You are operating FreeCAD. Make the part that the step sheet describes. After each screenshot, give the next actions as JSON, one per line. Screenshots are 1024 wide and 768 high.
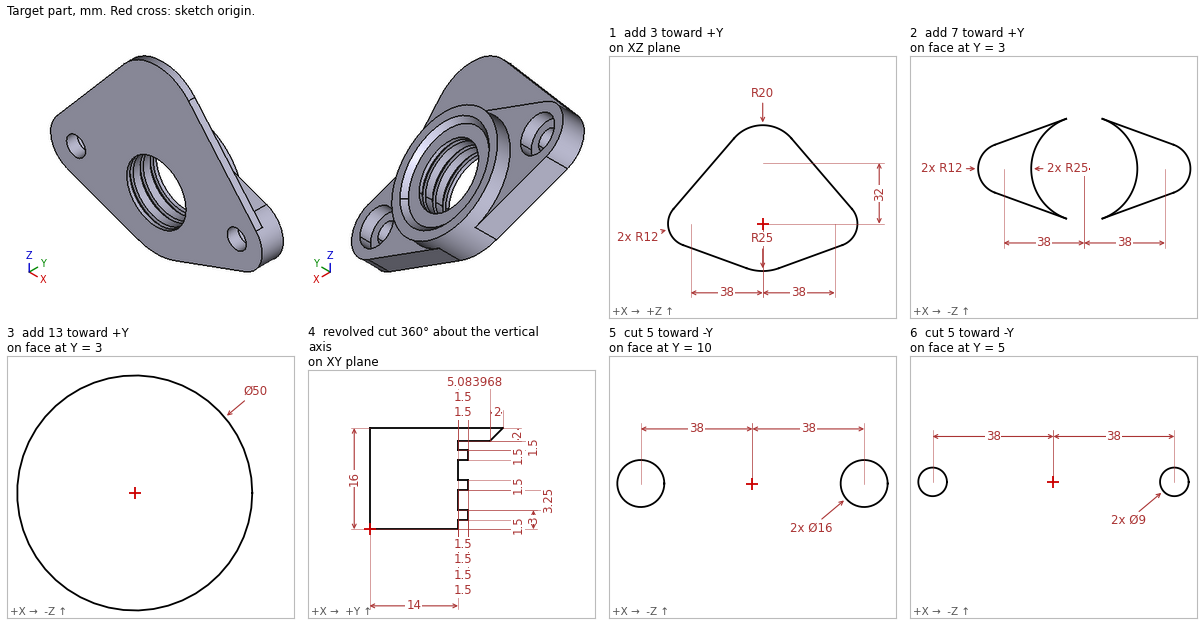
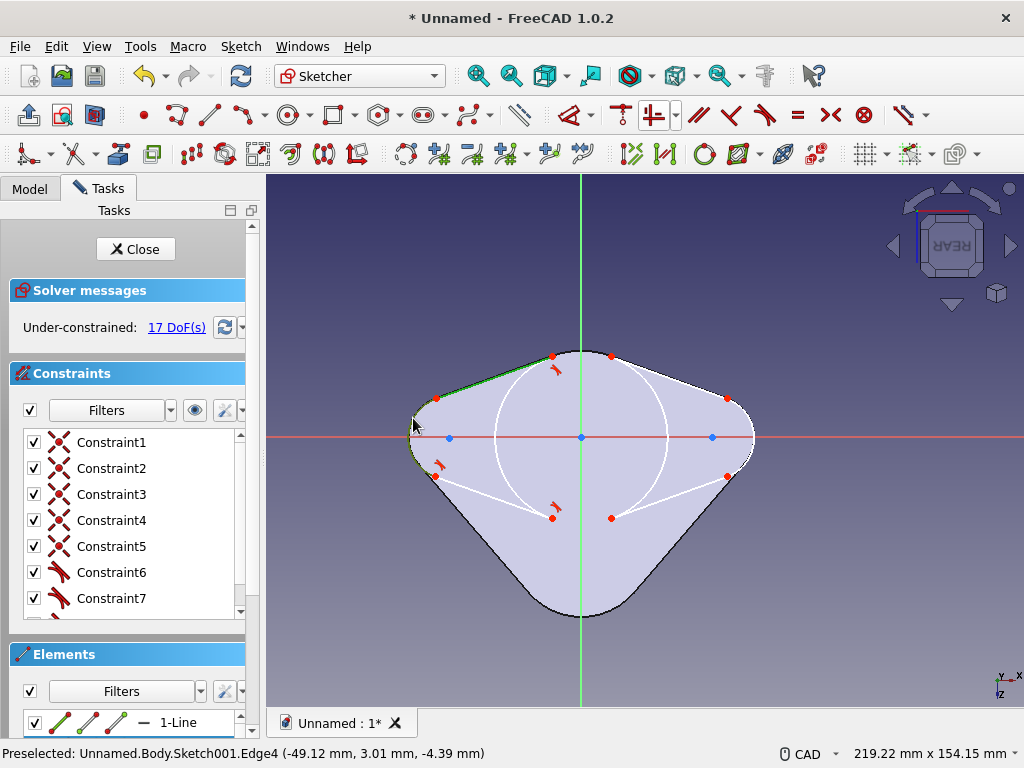
{"action": "left_click", "coordinate": [765, 116]}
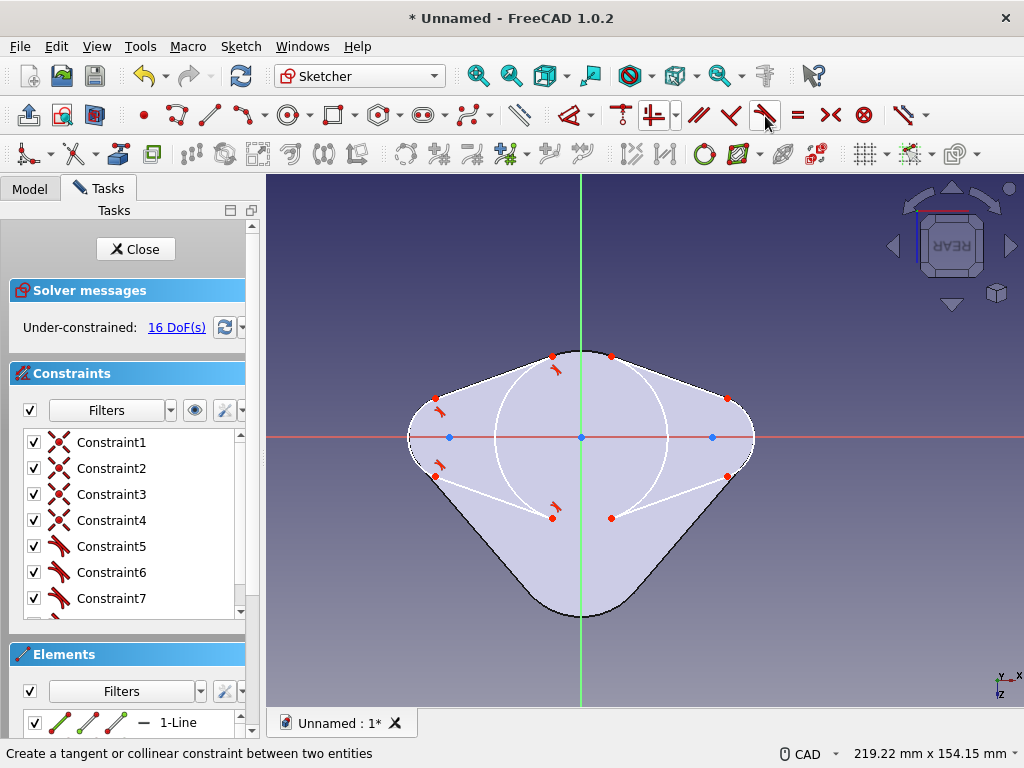
{"action": "left_click", "coordinate": [692, 490]}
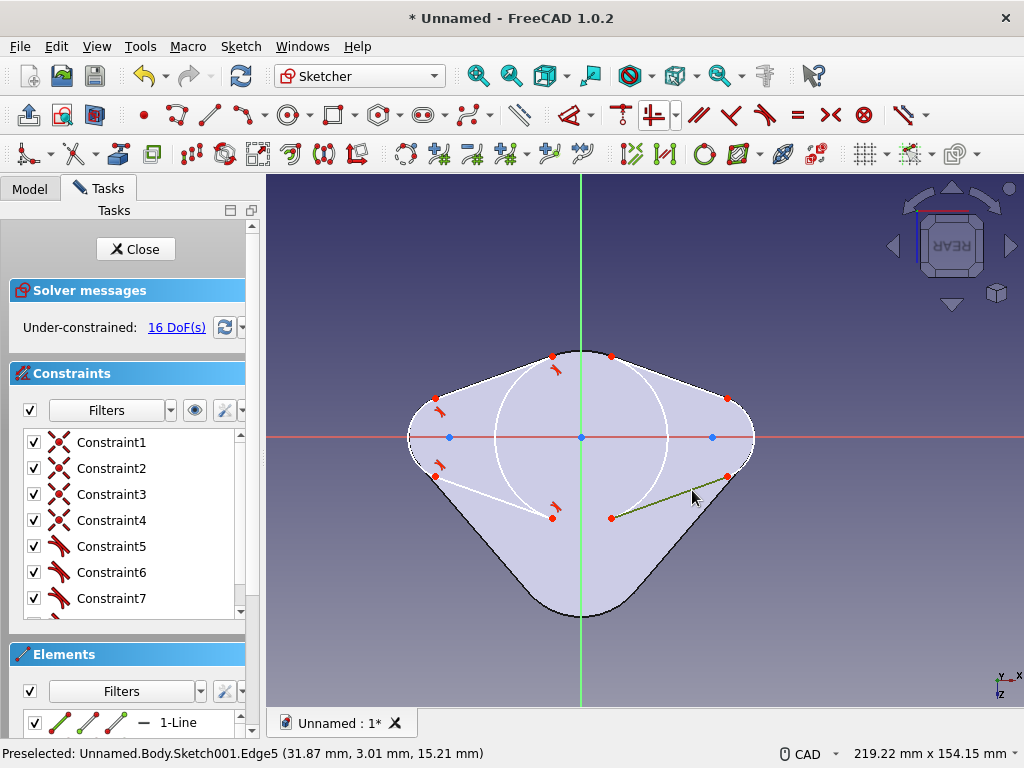
{"action": "left_click", "coordinate": [749, 457]}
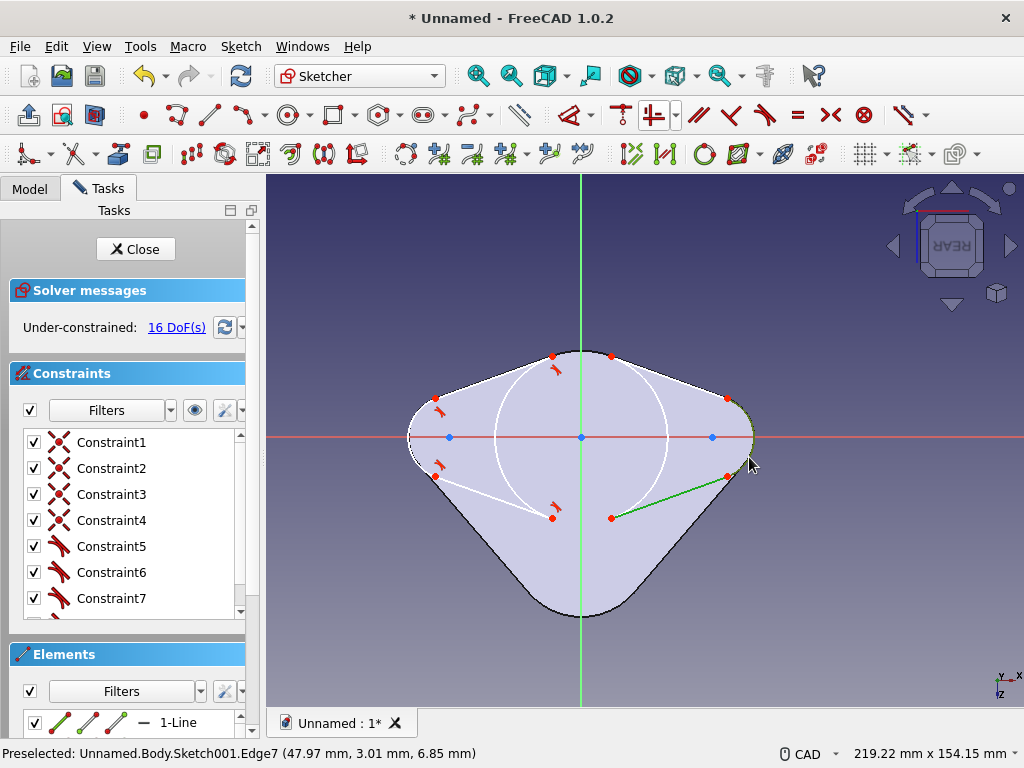
{"action": "left_click", "coordinate": [765, 116]}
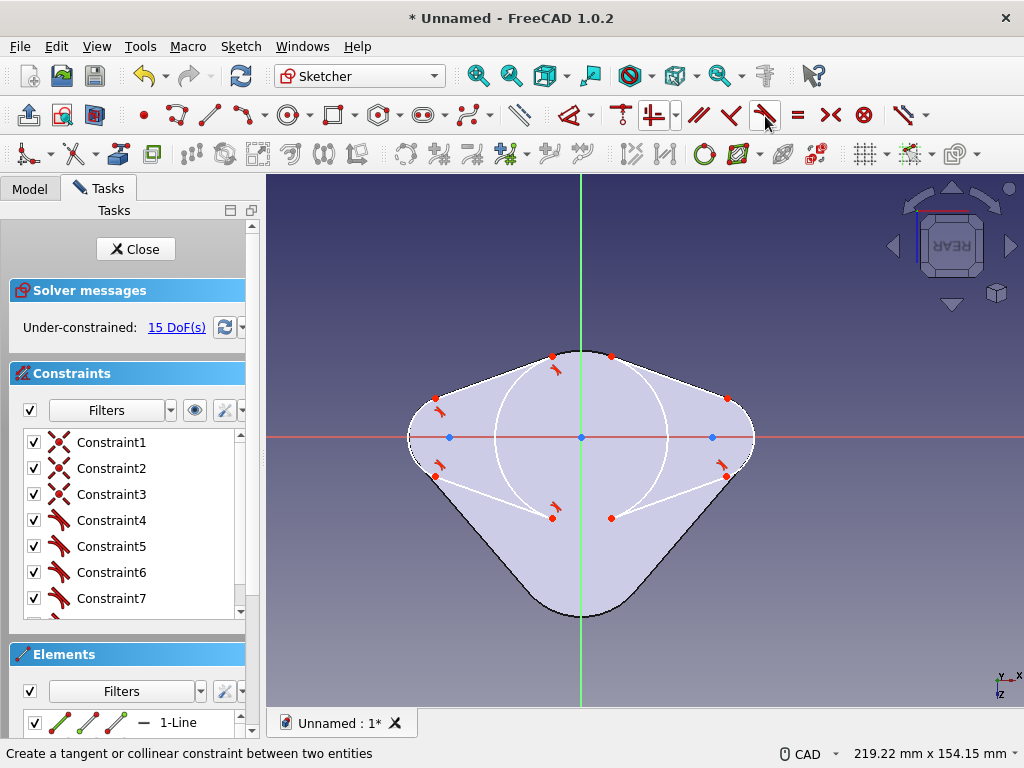
{"action": "left_click", "coordinate": [692, 490]}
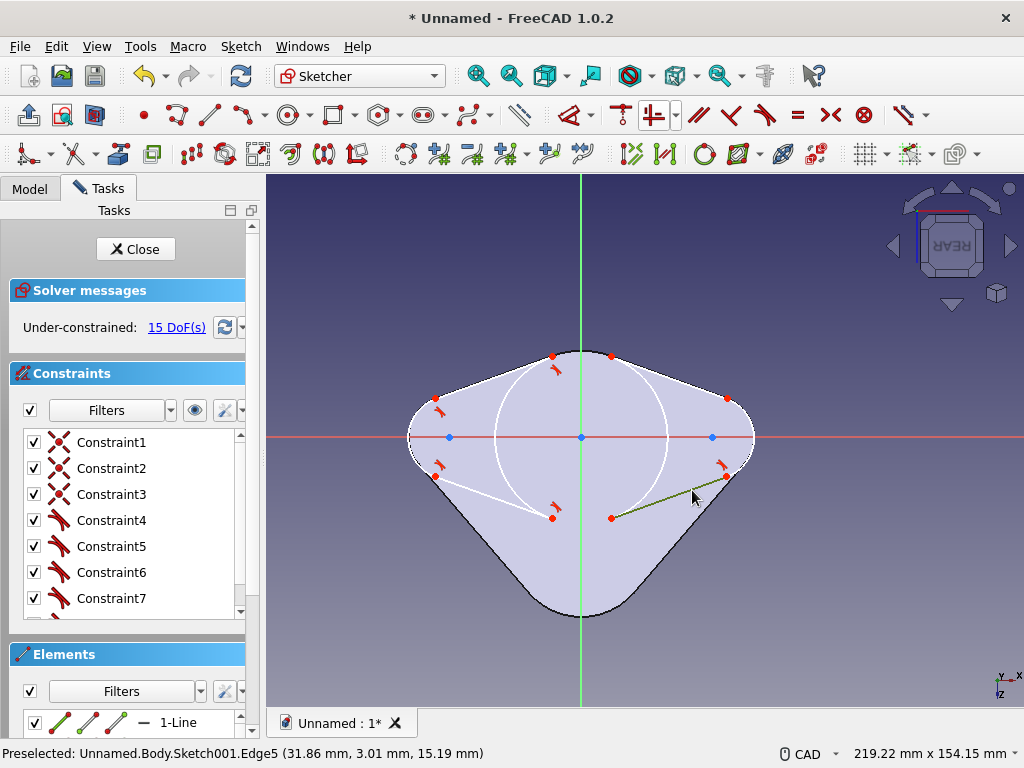
{"action": "left_click", "coordinate": [658, 478]}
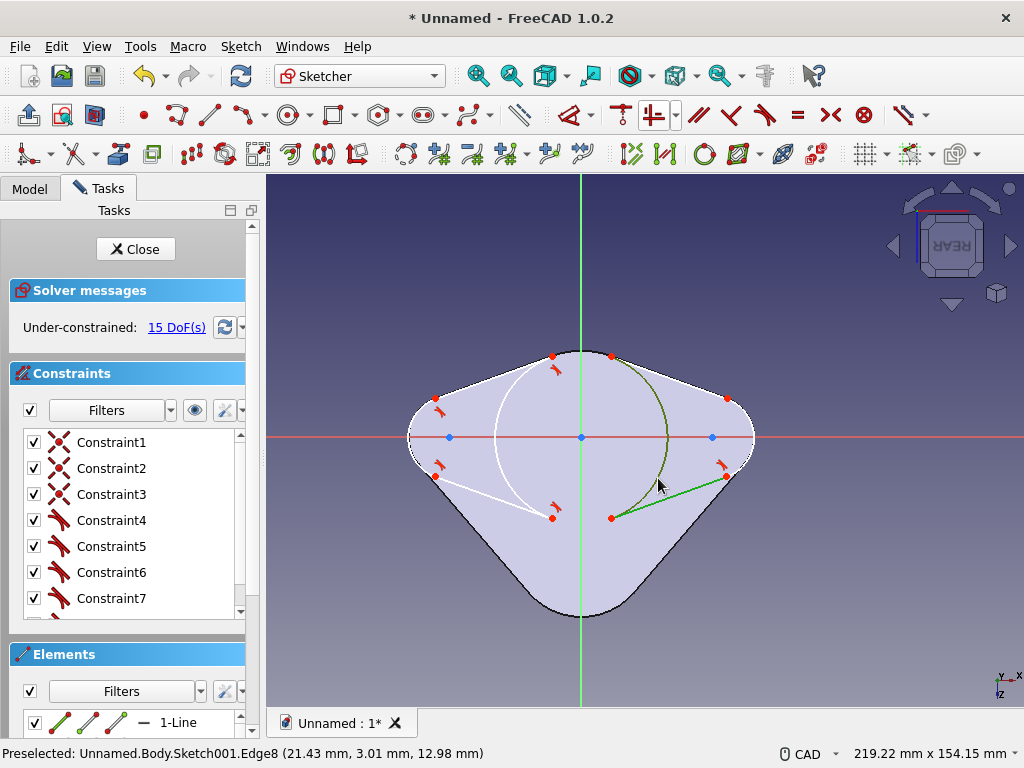
{"action": "left_click", "coordinate": [765, 116]}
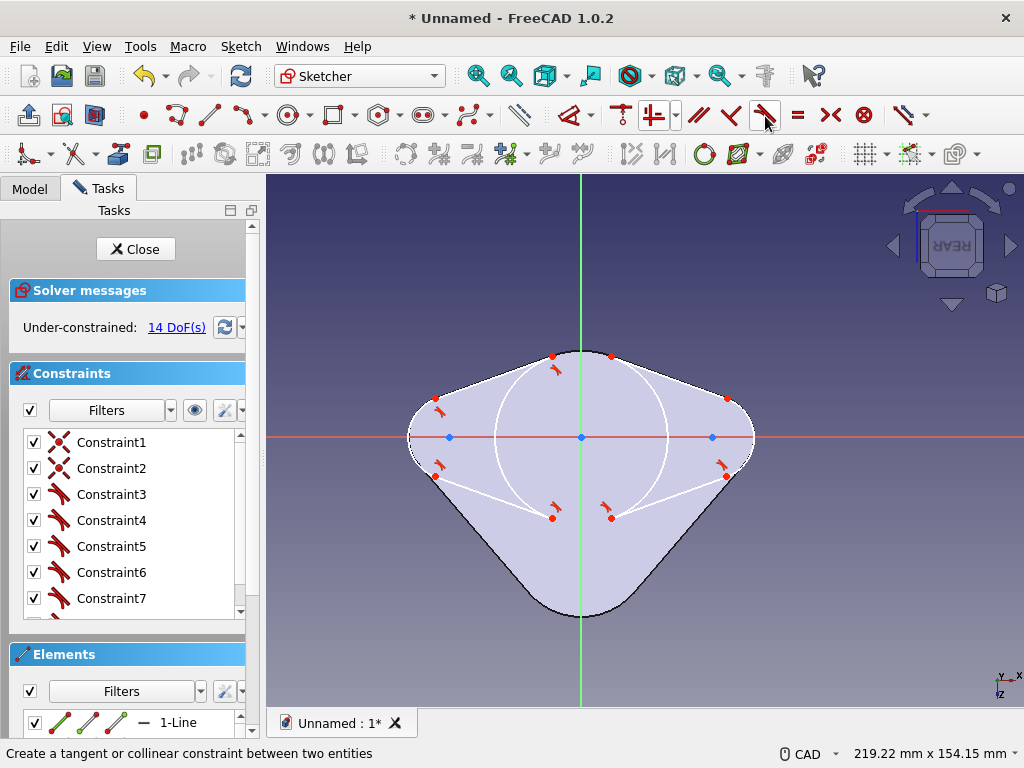
{"action": "left_click", "coordinate": [692, 386]}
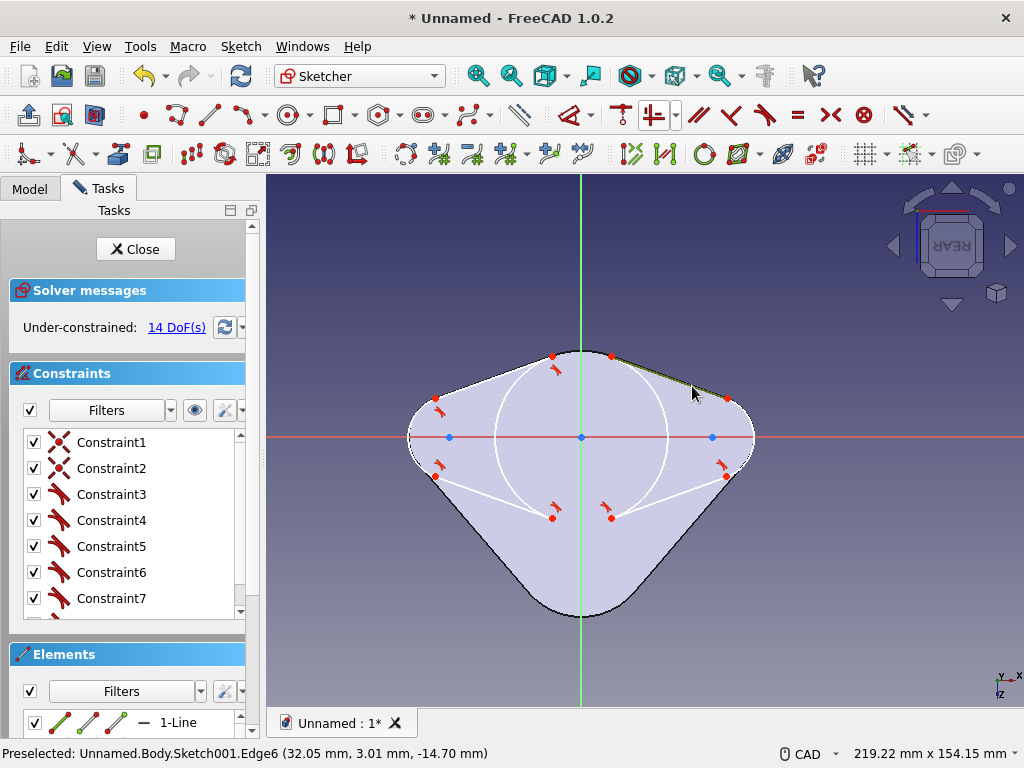
{"action": "left_click", "coordinate": [749, 458]}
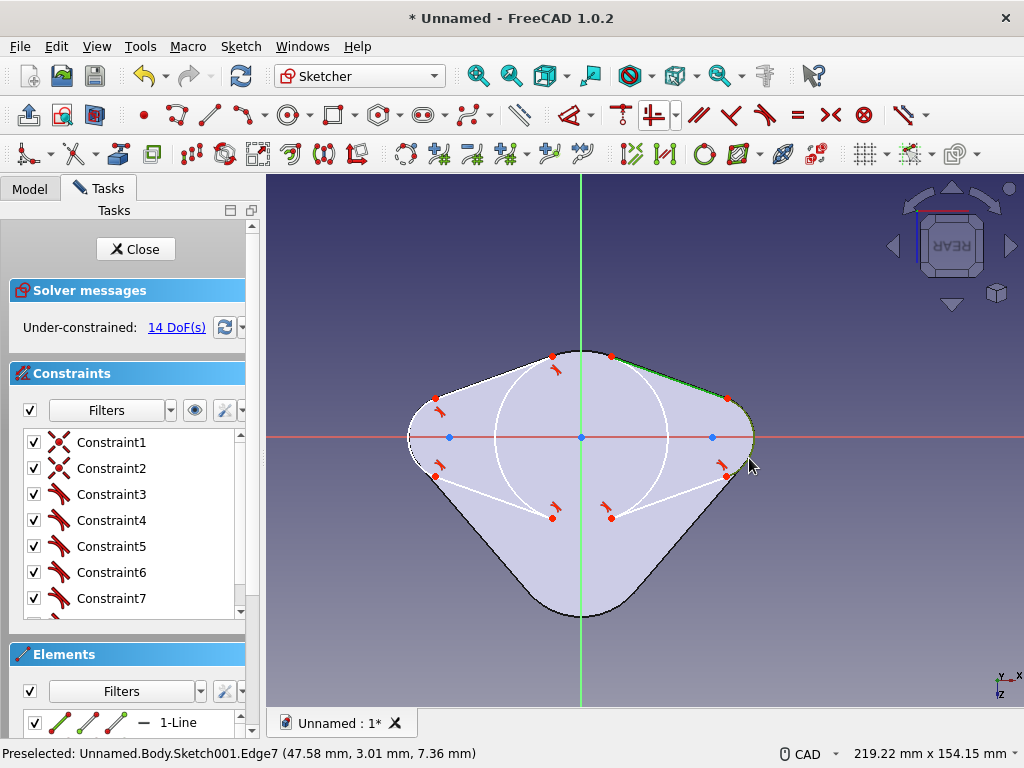
{"action": "left_click", "coordinate": [765, 116]}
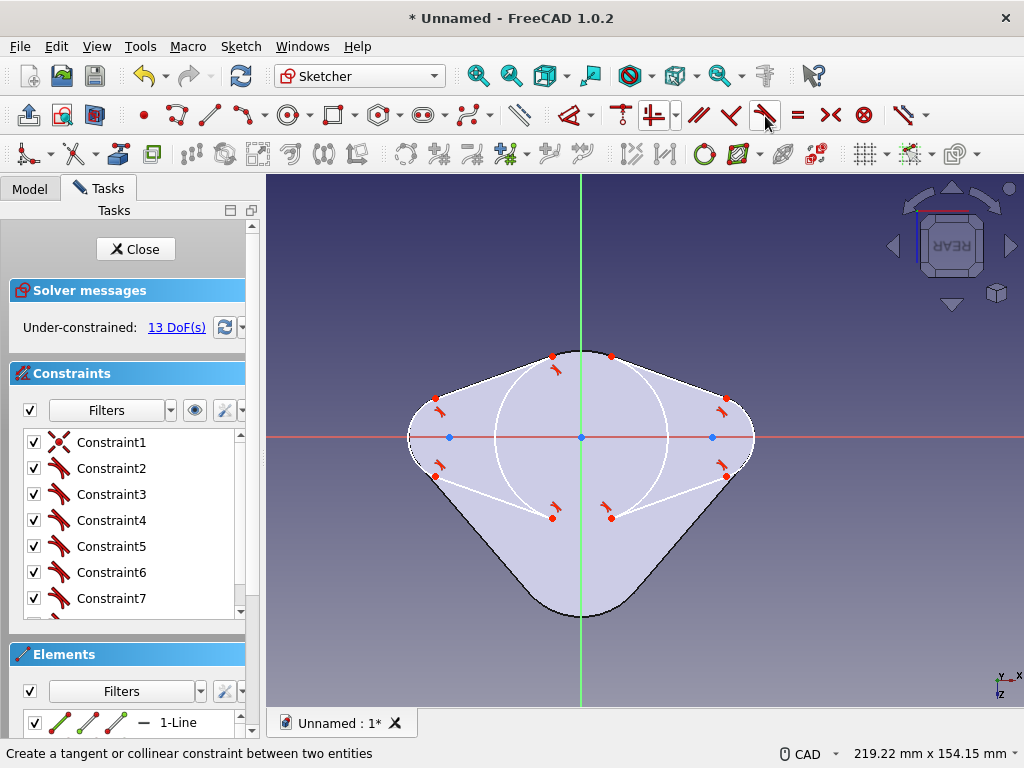
{"action": "left_click", "coordinate": [692, 386]}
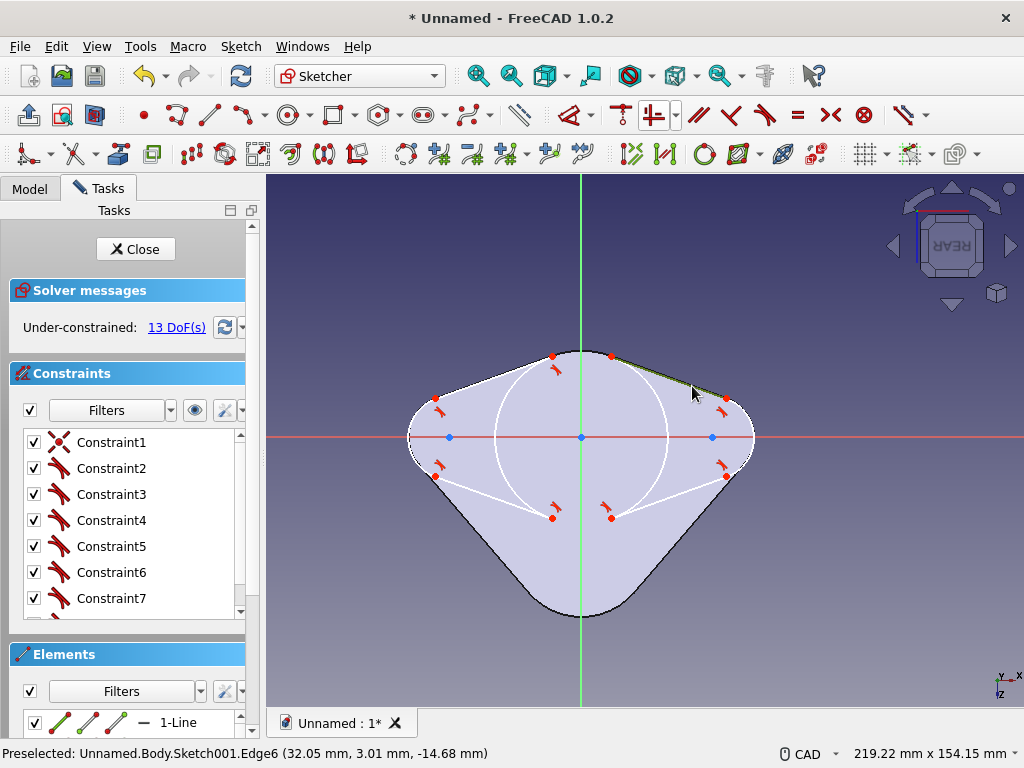
{"action": "left_click", "coordinate": [658, 478]}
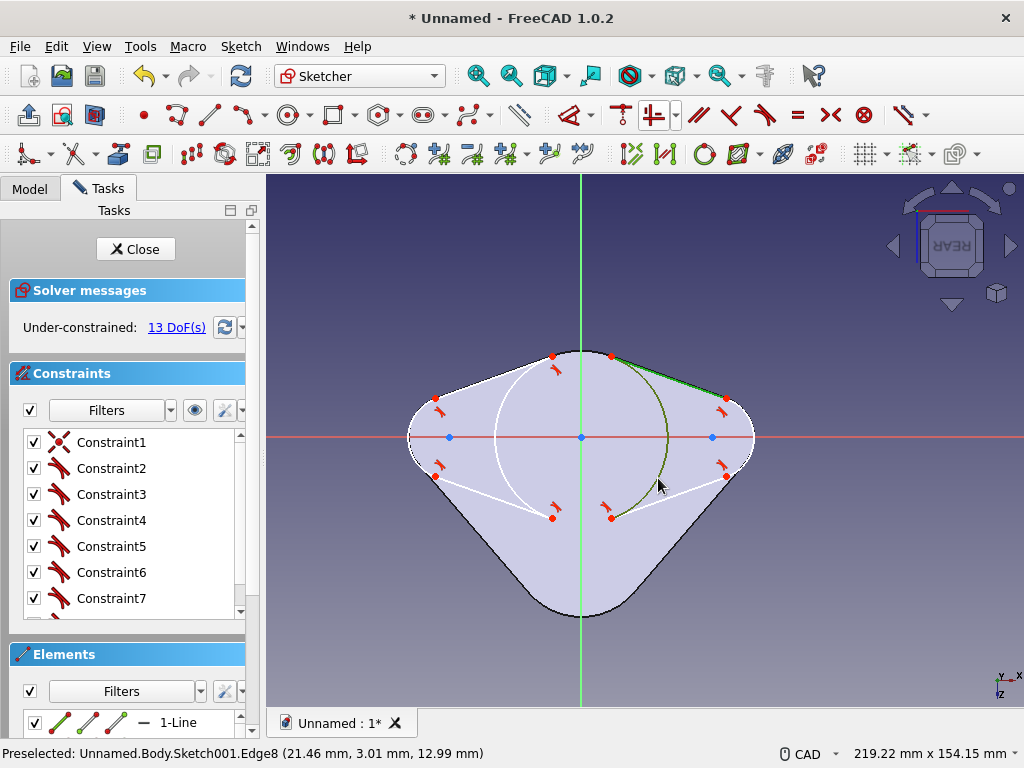
{"action": "left_click", "coordinate": [765, 116]}